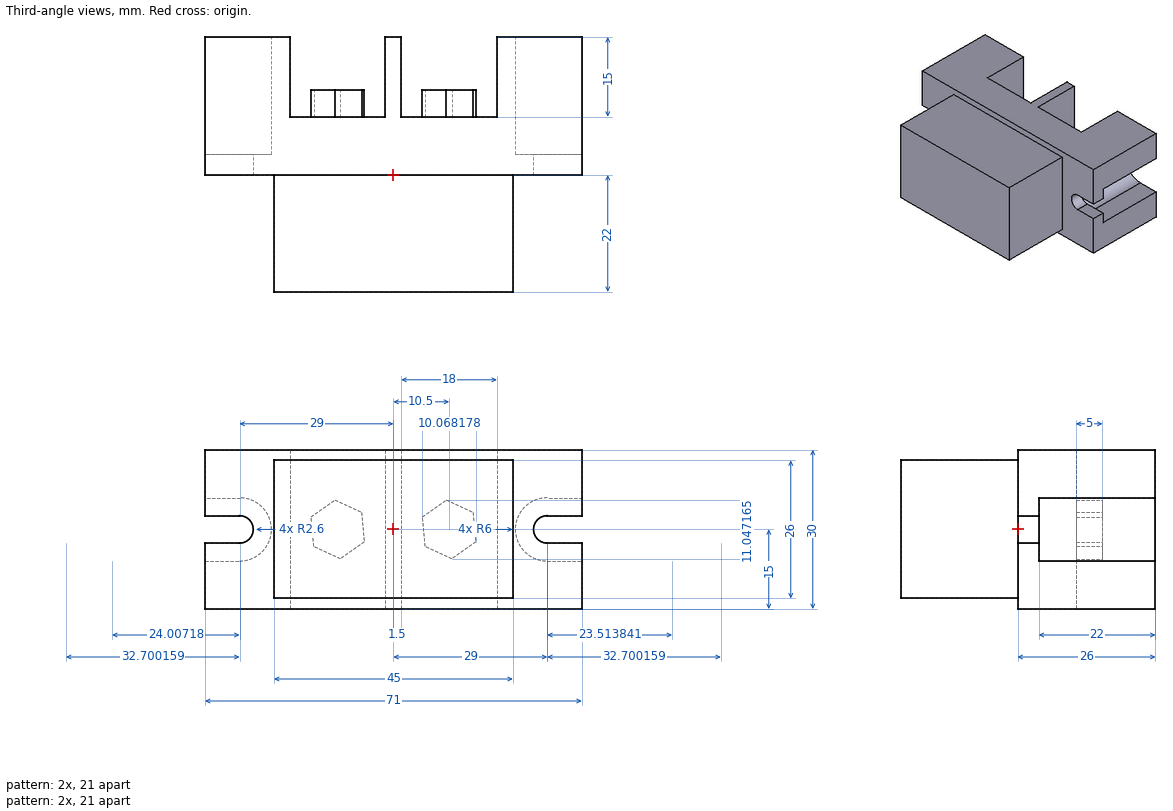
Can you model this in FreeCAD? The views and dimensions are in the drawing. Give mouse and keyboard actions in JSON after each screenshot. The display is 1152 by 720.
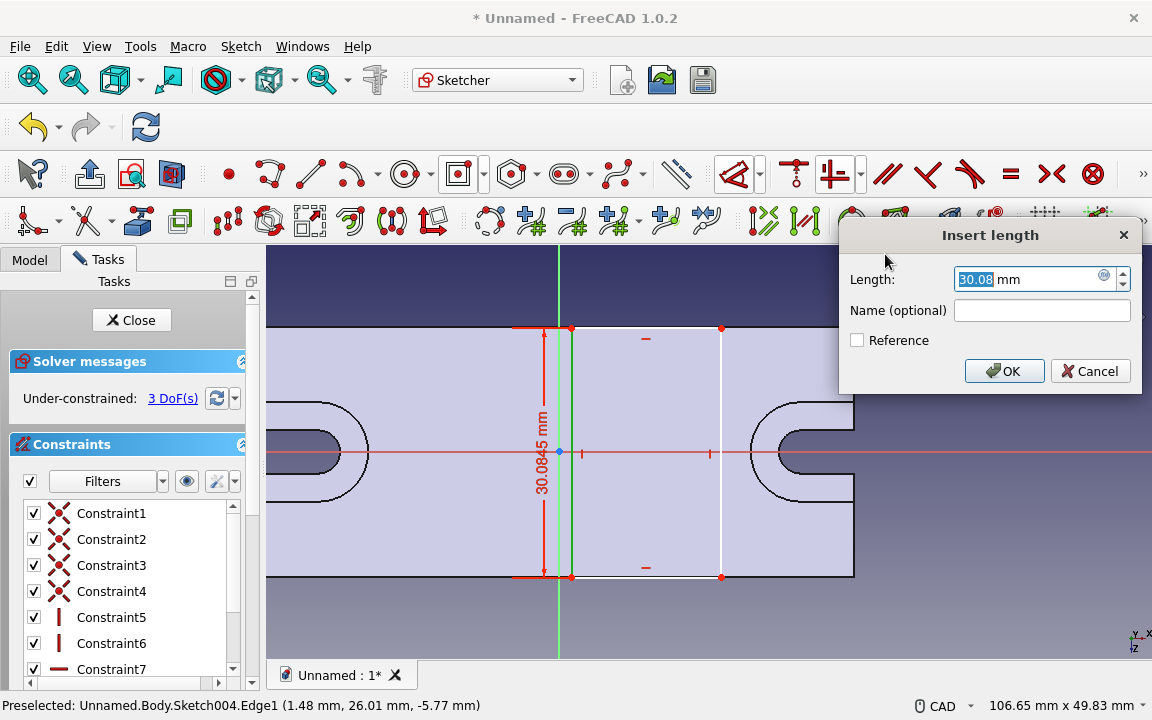
{"action": "type", "text": "30"}
{"action": "key", "text": "Return"}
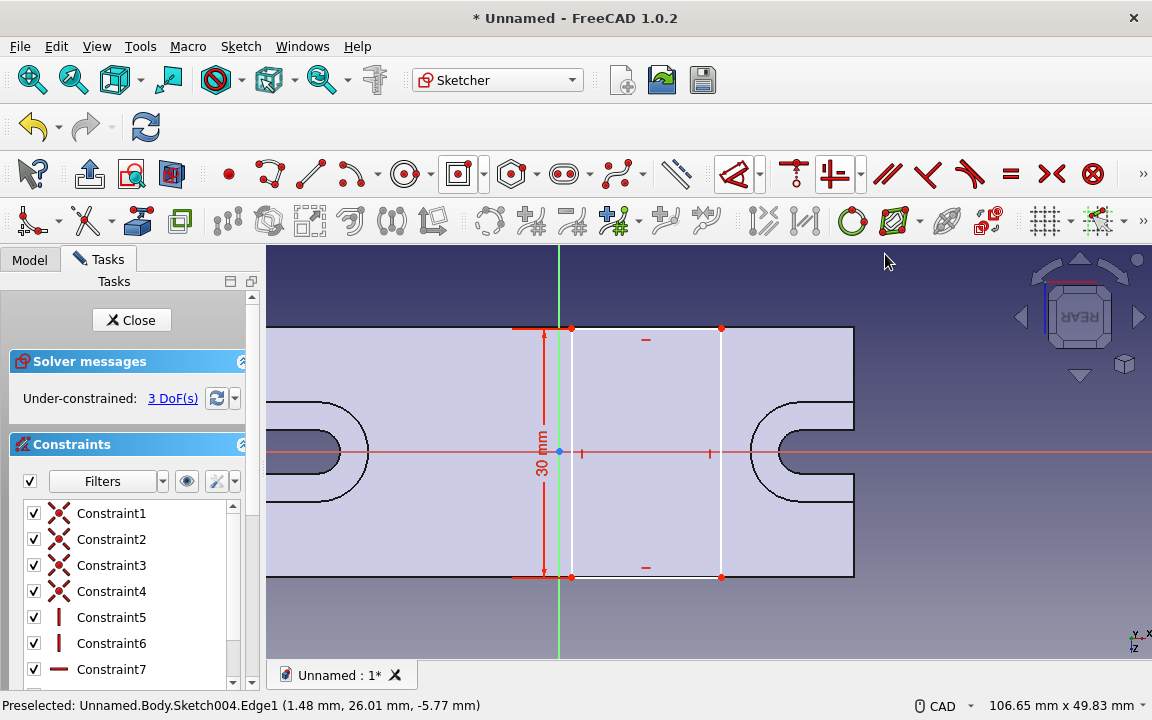
{"action": "left_click", "coordinate": [617, 578]}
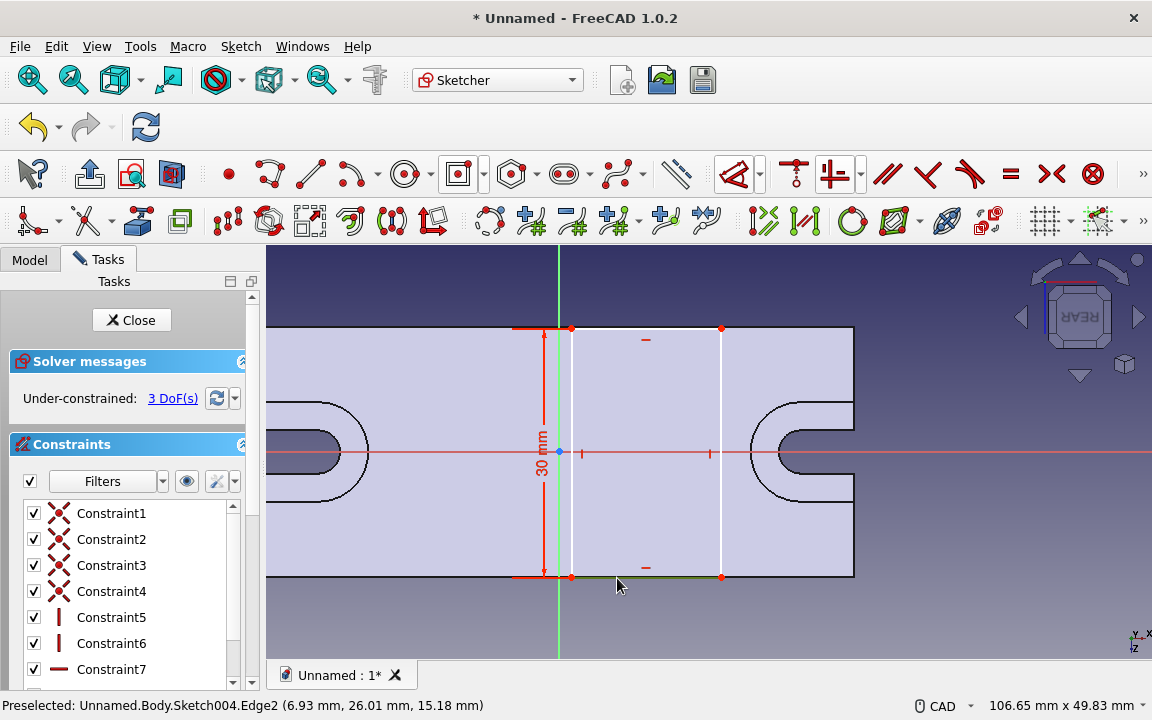
{"action": "left_click", "coordinate": [760, 174]}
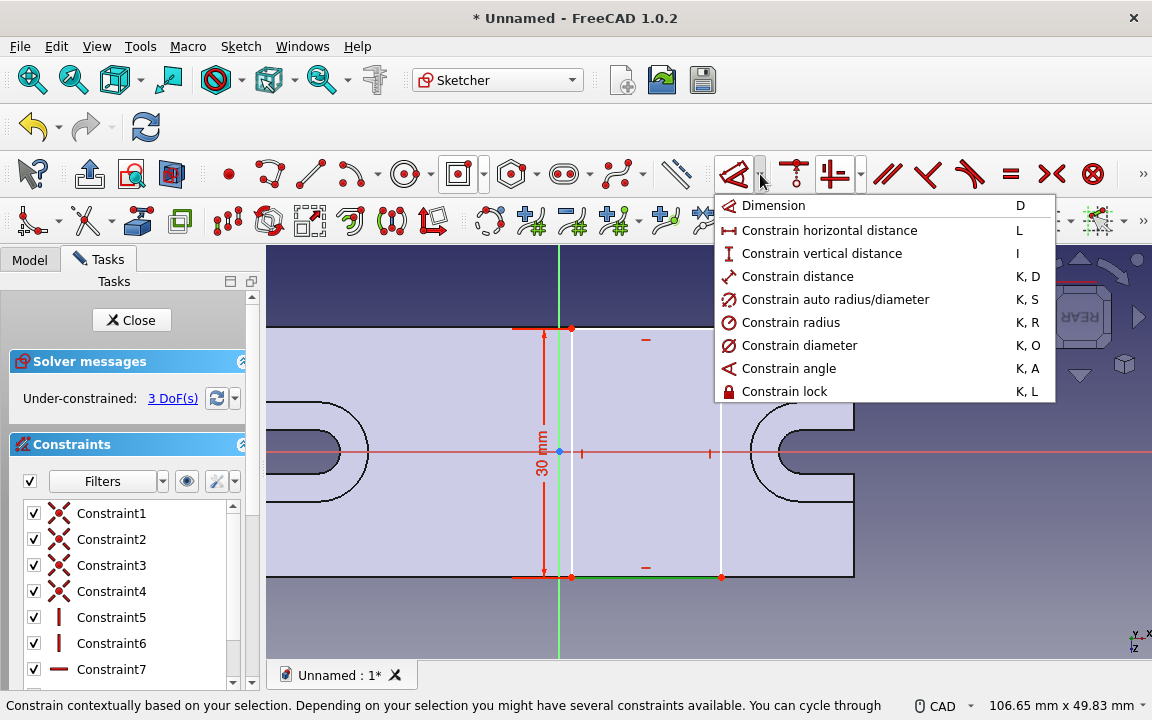
{"action": "left_click", "coordinate": [885, 230]}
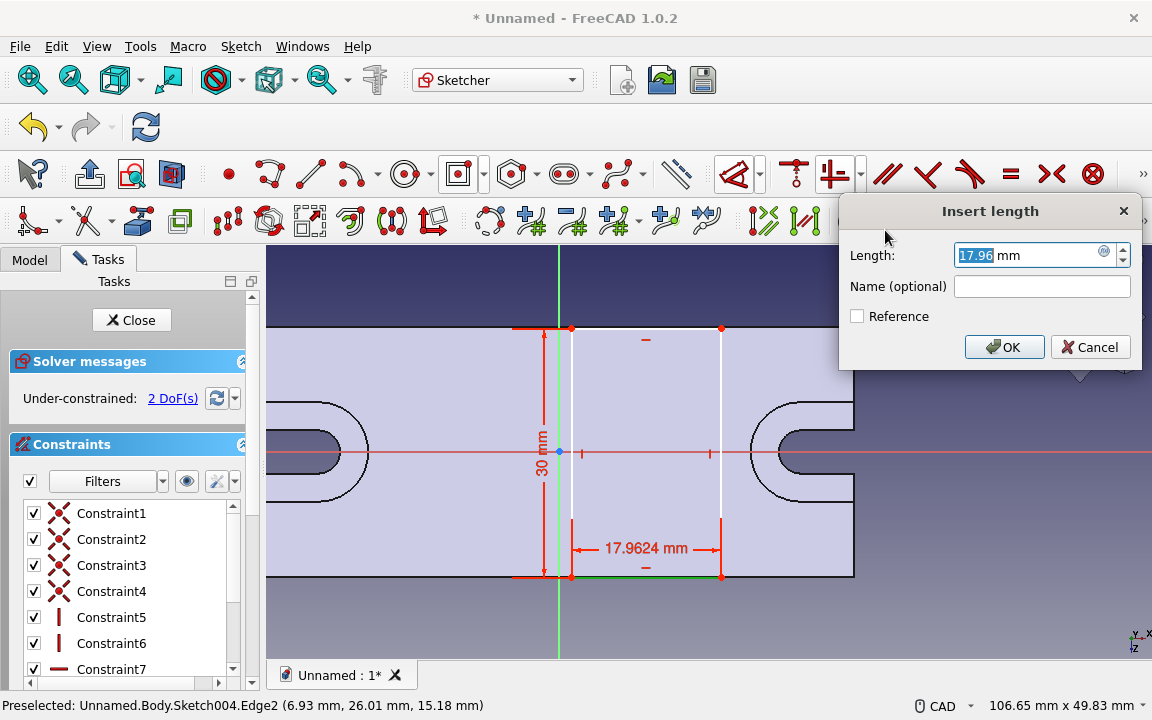
{"action": "type", "text": "18"}
{"action": "key", "text": "Return"}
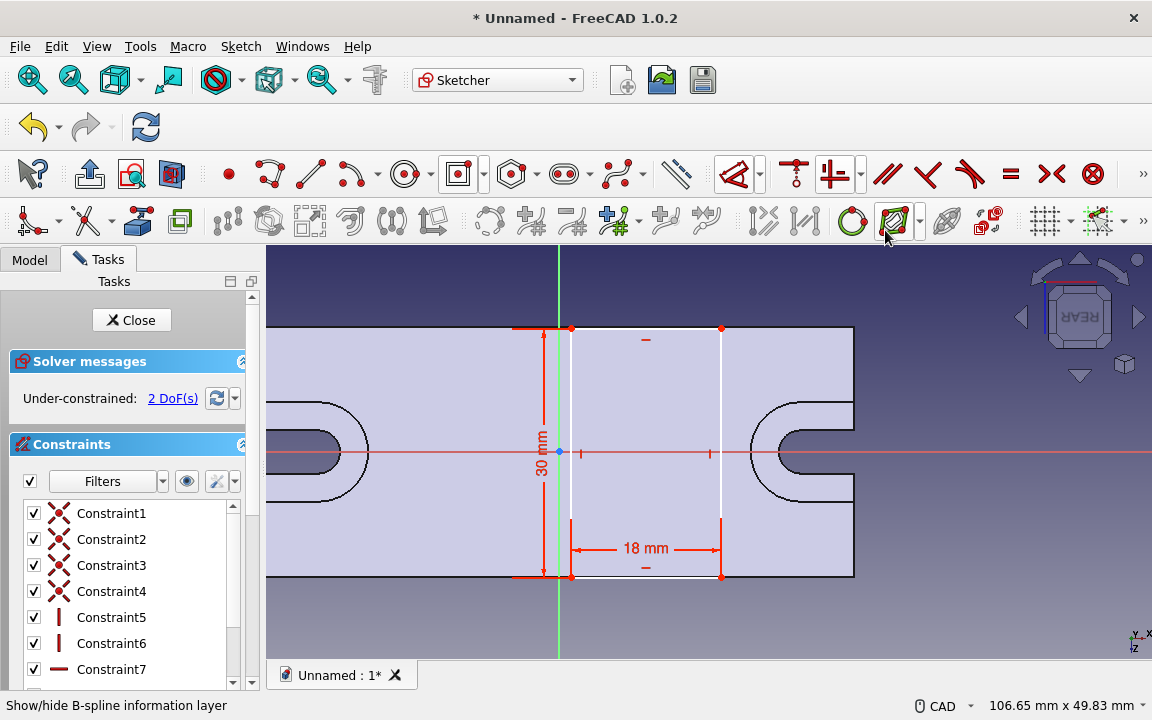
{"action": "left_click", "coordinate": [571, 329]}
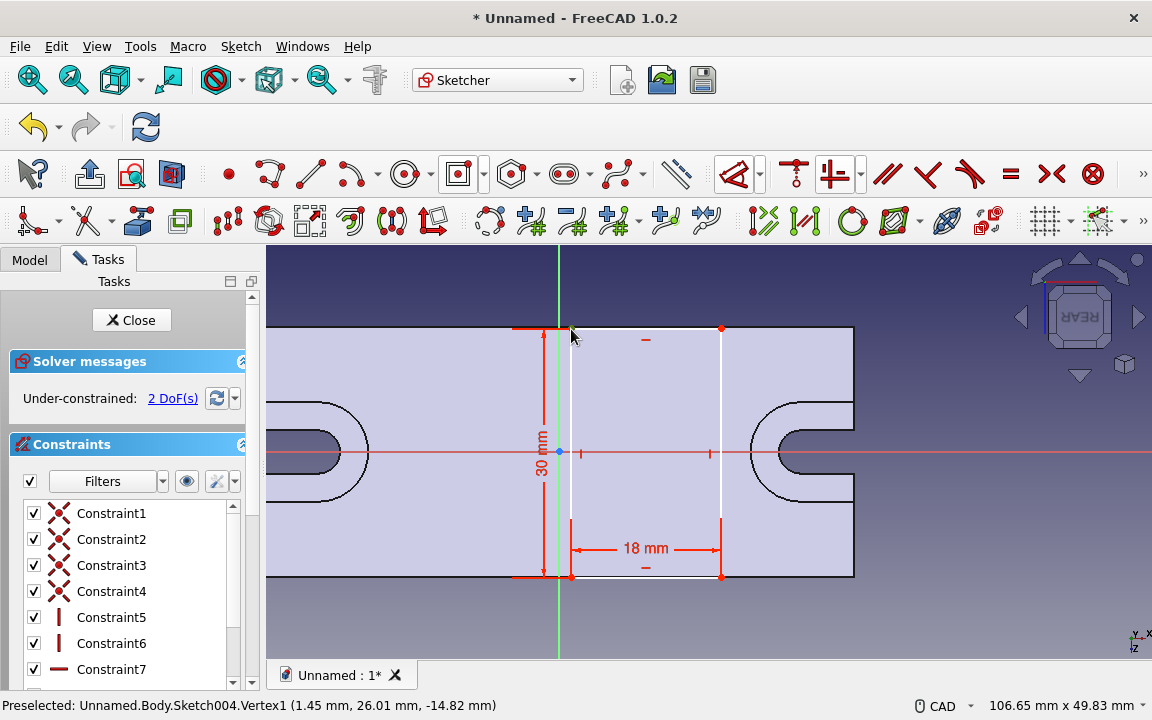
{"action": "left_click", "coordinate": [760, 174]}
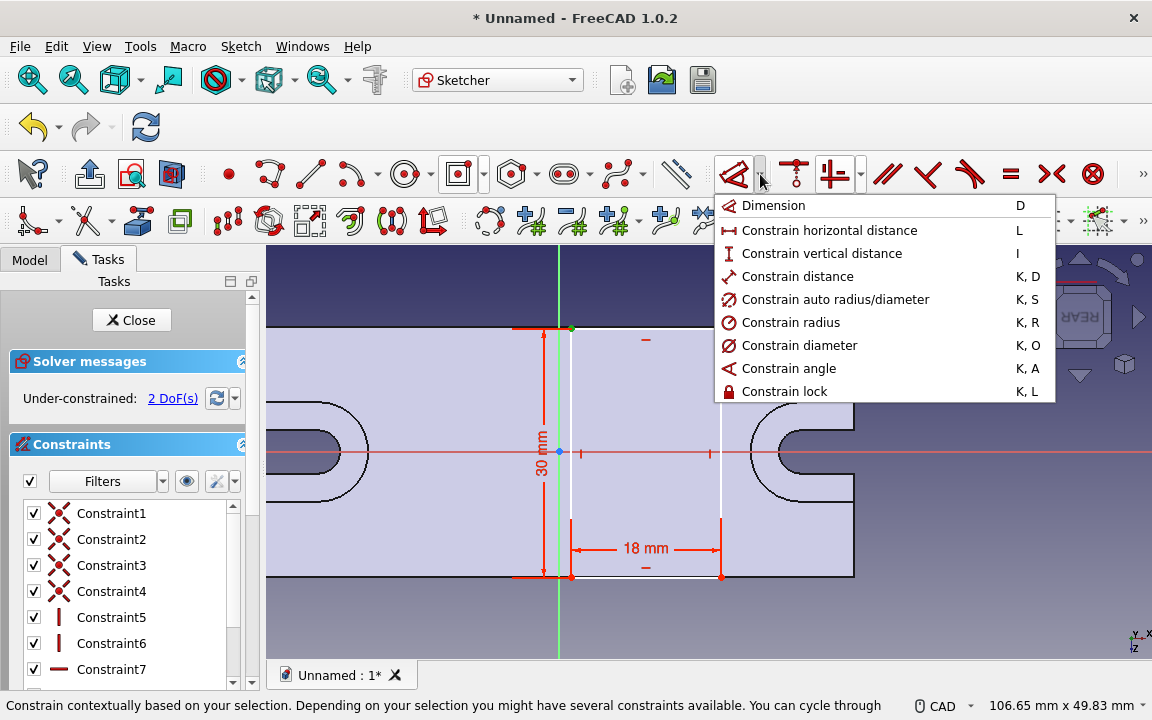
{"action": "left_click", "coordinate": [885, 254]}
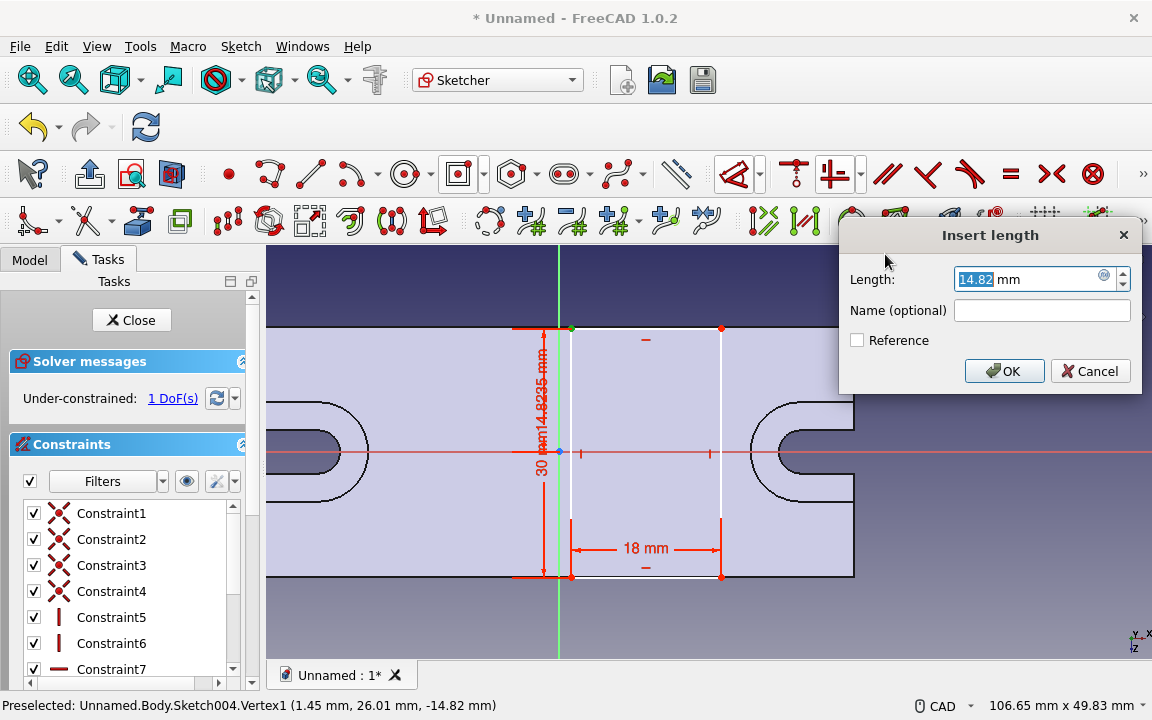
{"action": "type", "text": "15"}
{"action": "key", "text": "Return"}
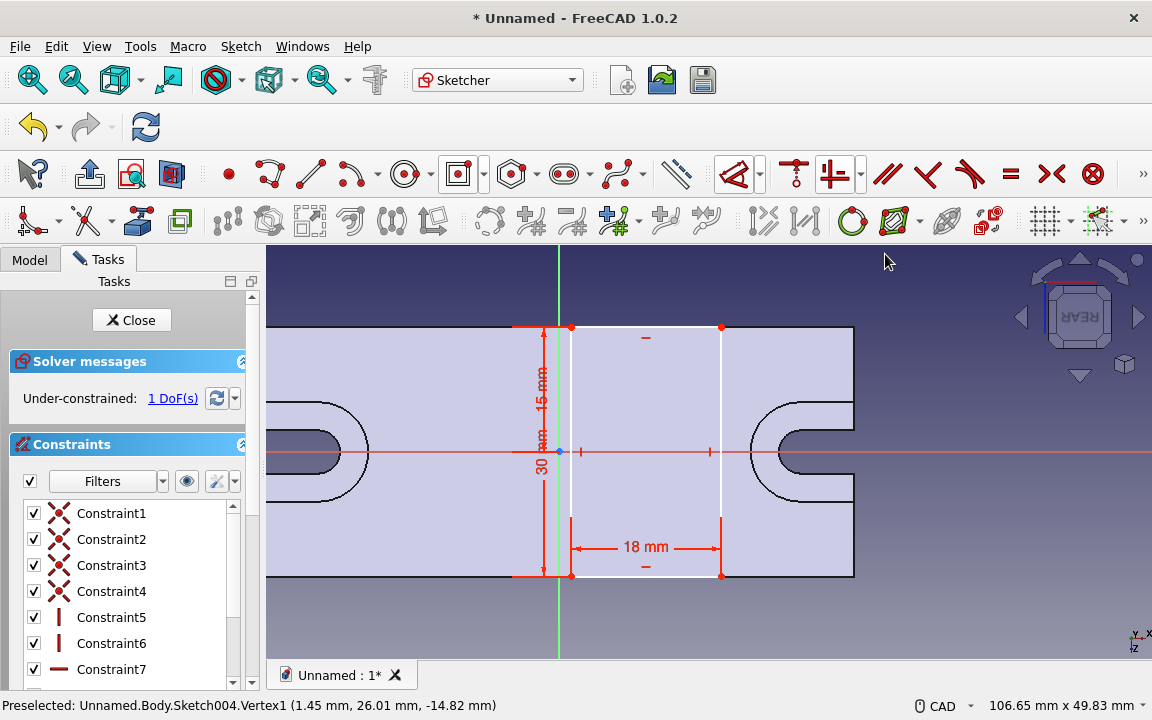
{"action": "scroll", "coordinate": [571, 327], "scroll_direction": "up", "scroll_amount": 6}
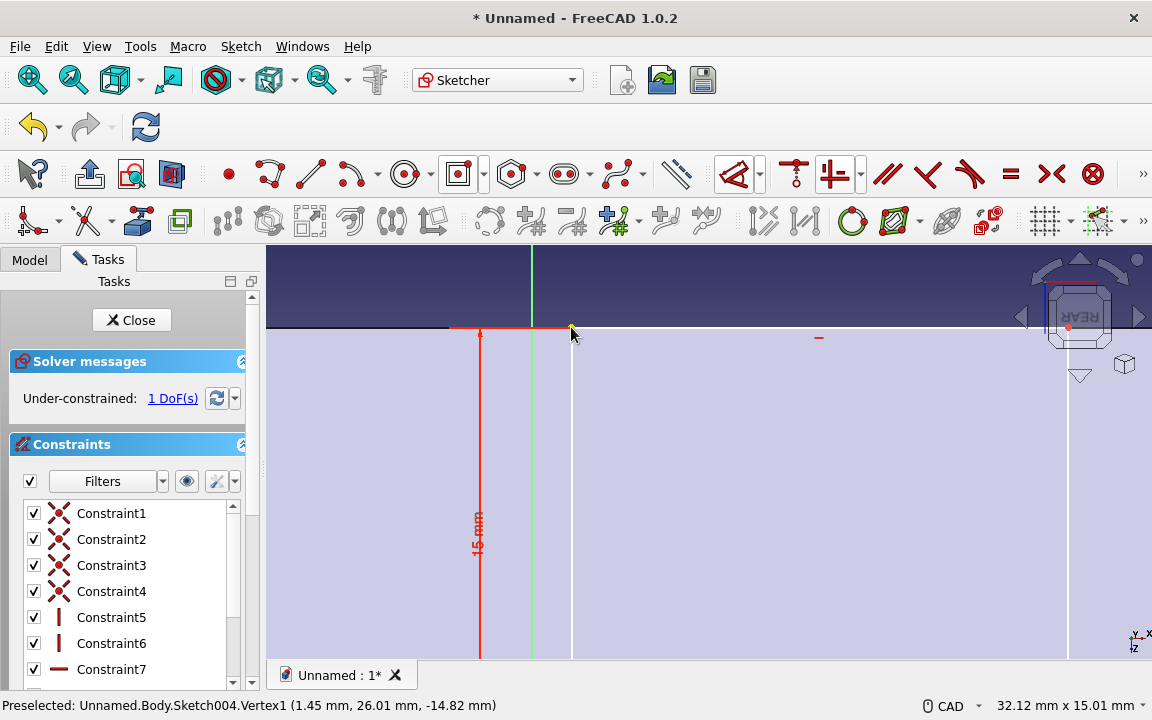
{"action": "left_click", "coordinate": [572, 328]}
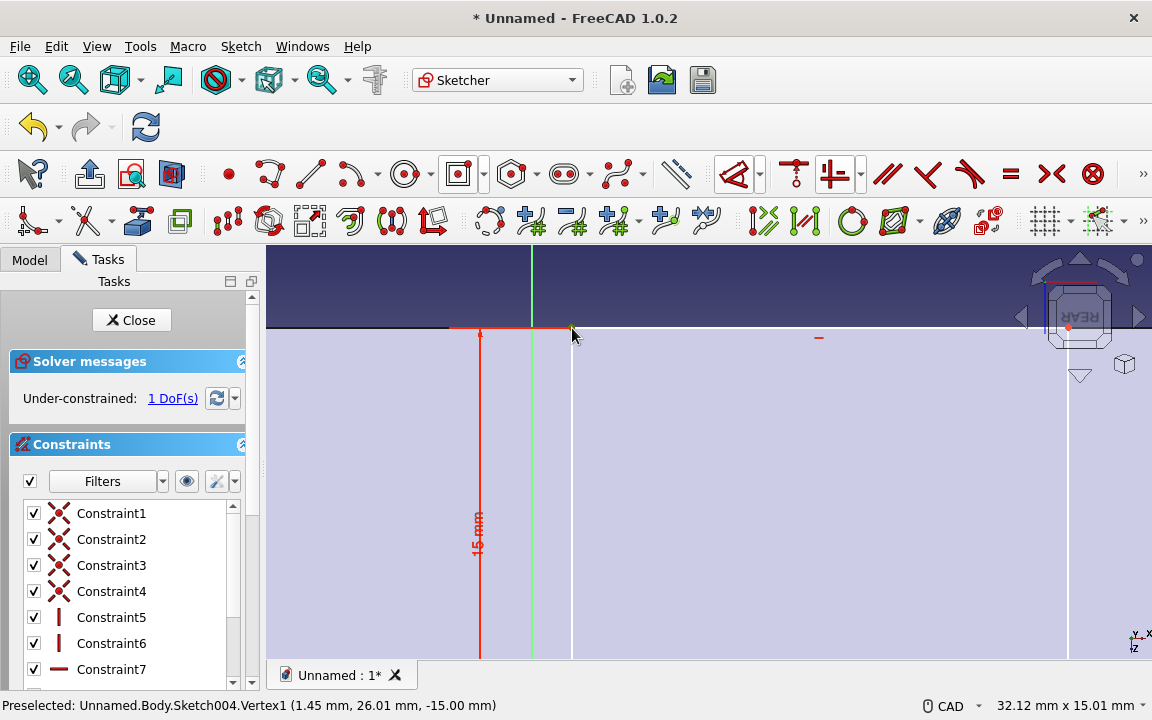
{"action": "left_click", "coordinate": [760, 174]}